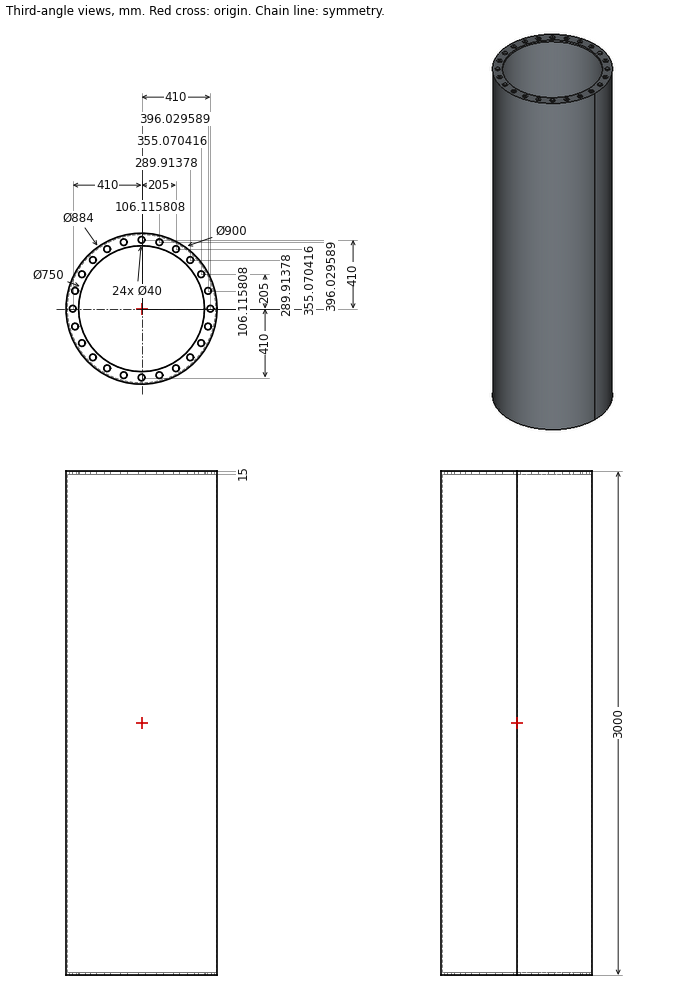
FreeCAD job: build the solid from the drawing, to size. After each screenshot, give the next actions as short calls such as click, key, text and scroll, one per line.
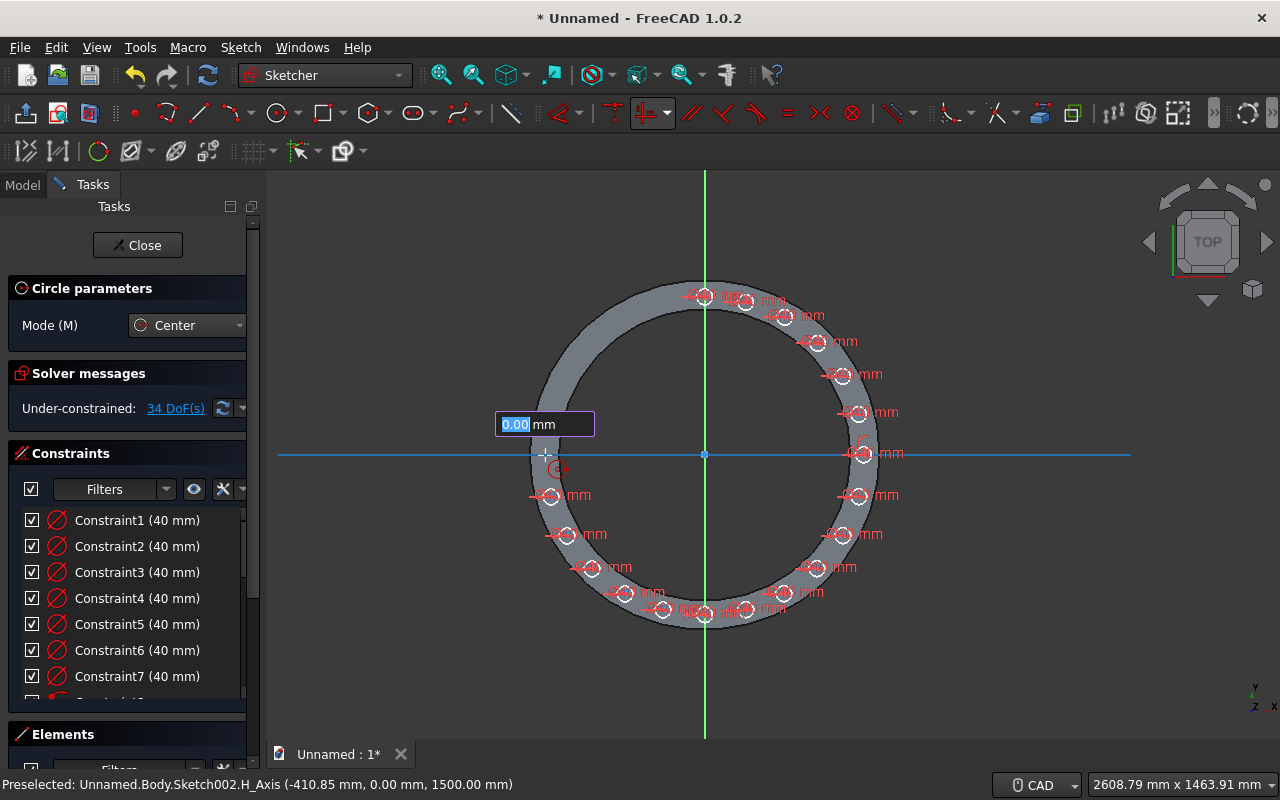
scroll(543, 462, up, 4)
move(542, 462)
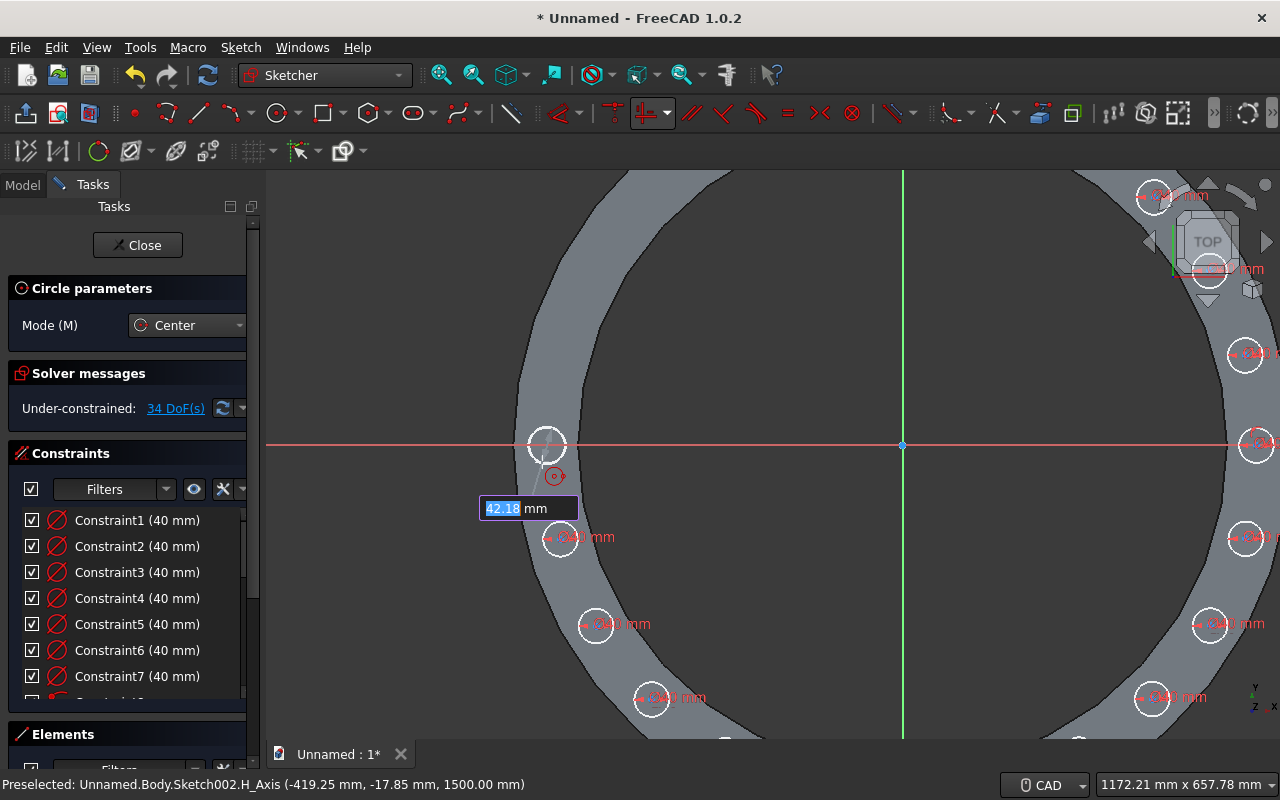
text(40)
key(Return)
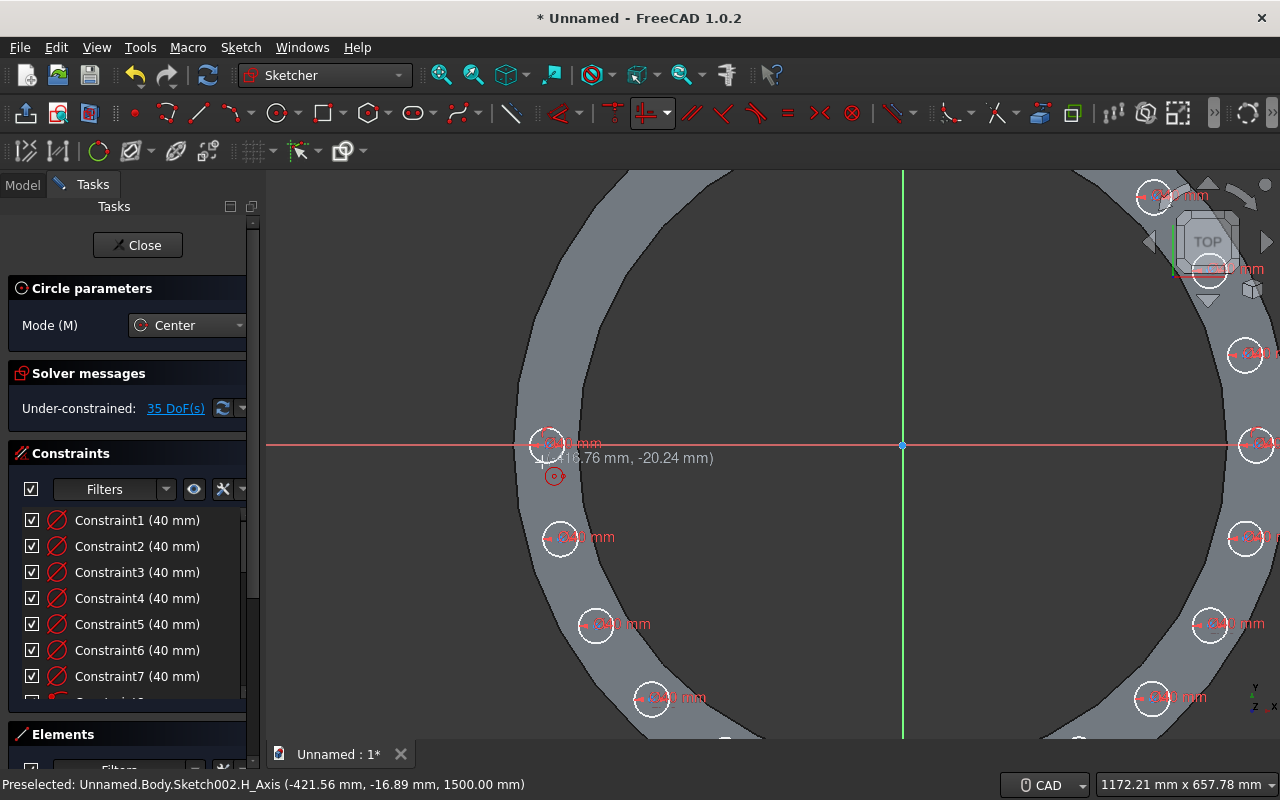
scroll(560, 354, up, 2)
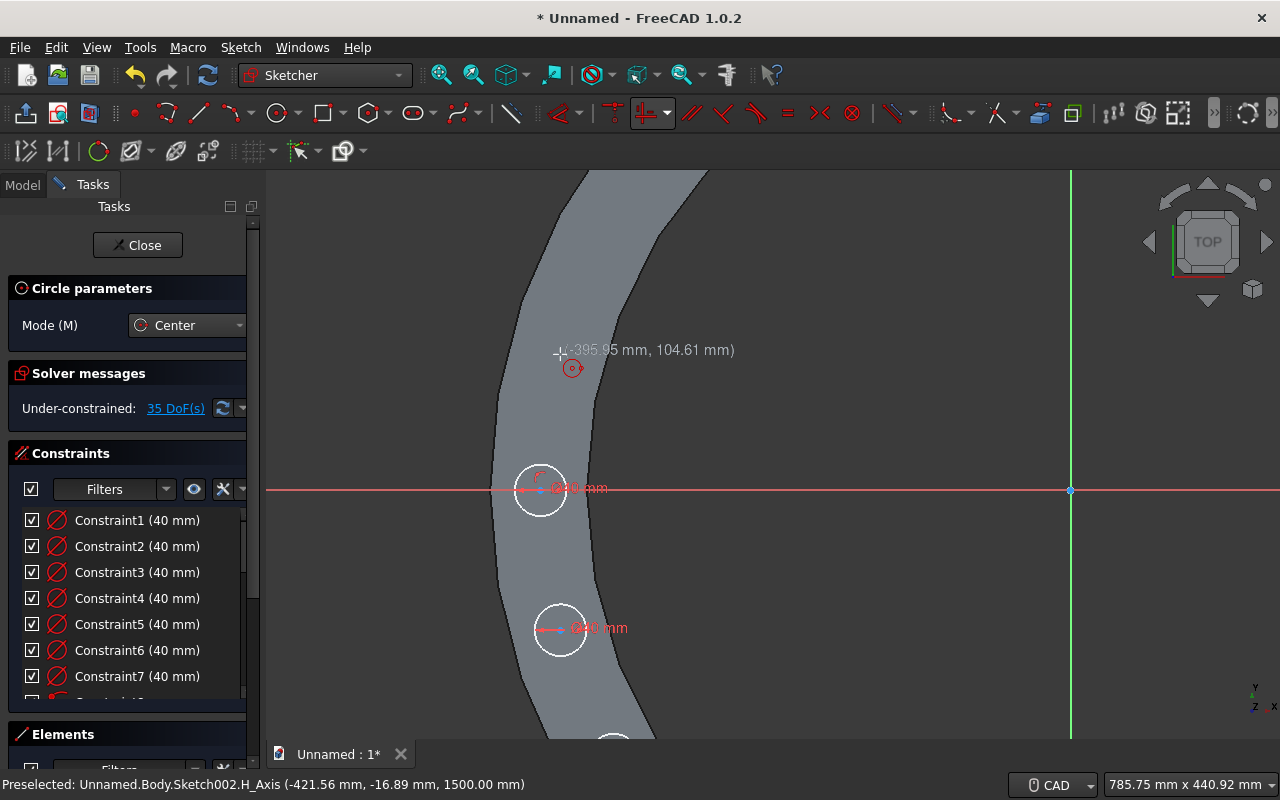
scroll(547, 439, down, 6)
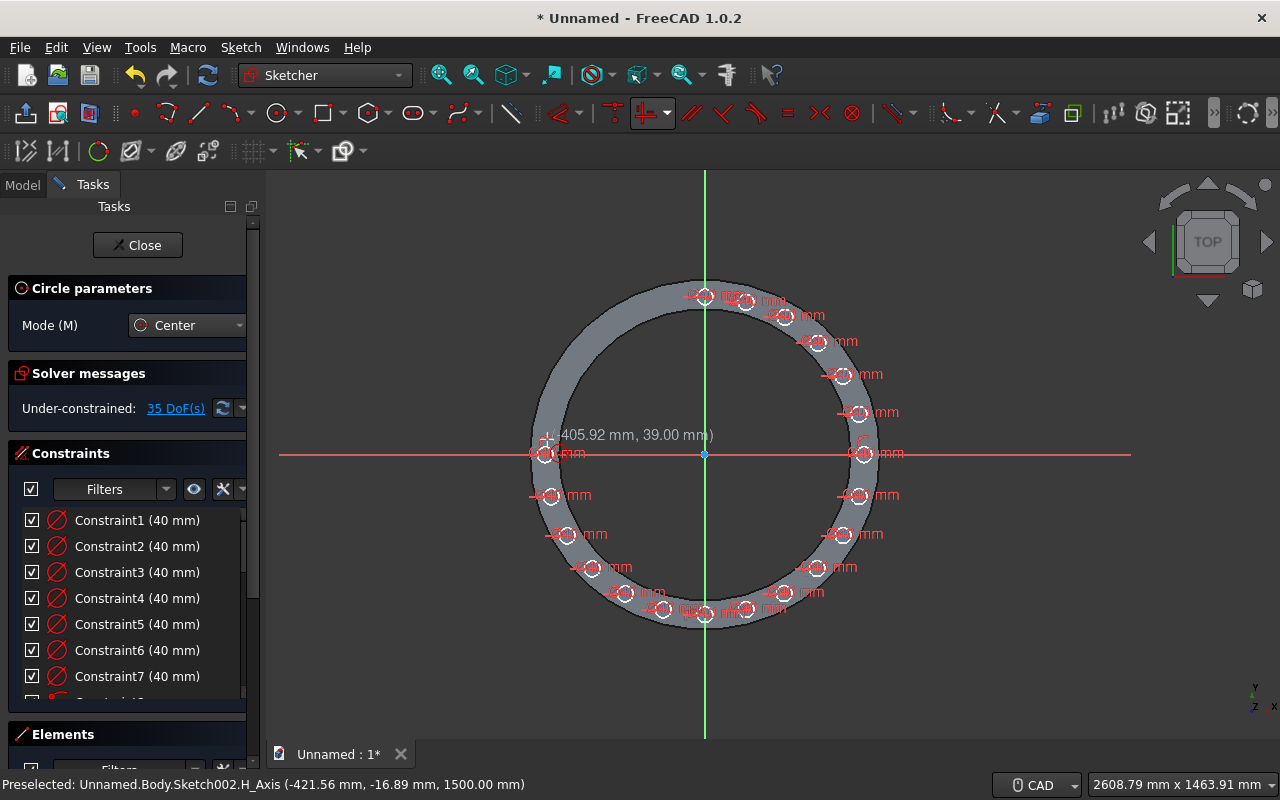
click(551, 414)
move(557, 408)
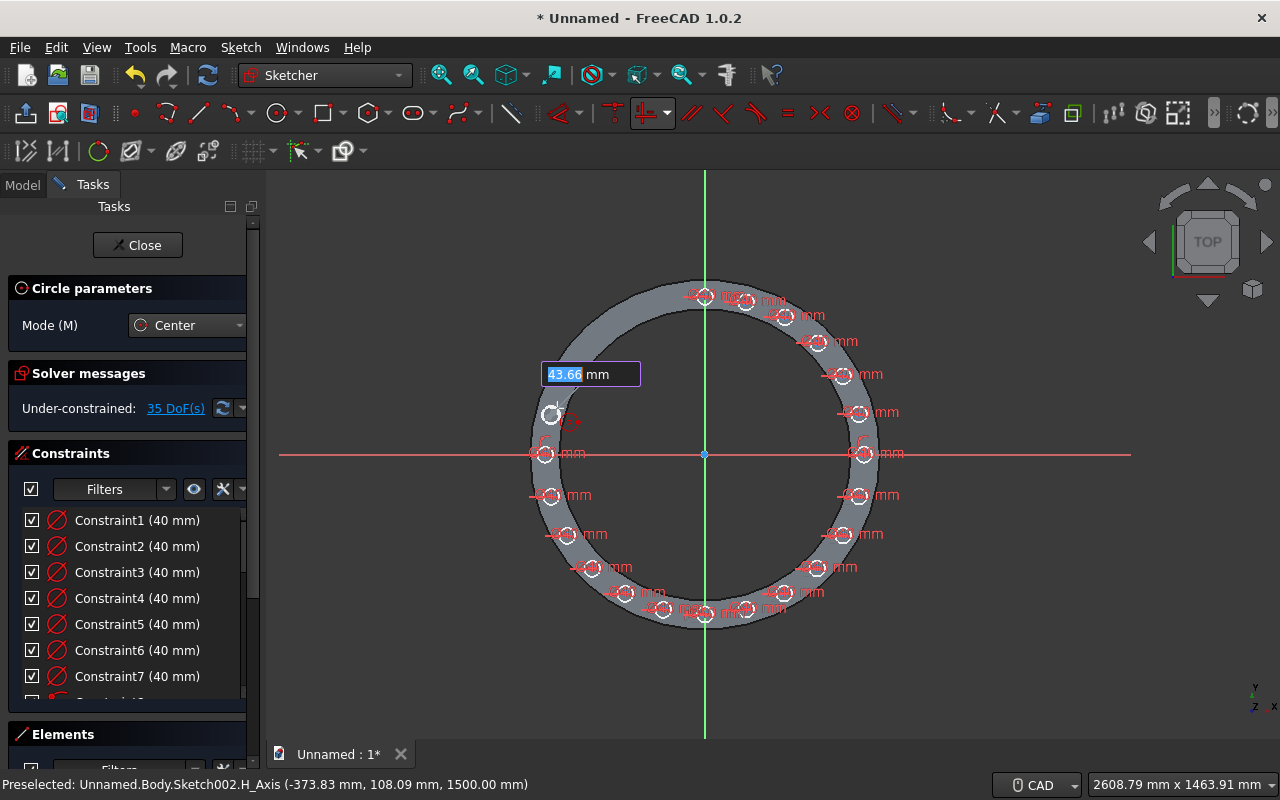
text(40)
key(Return)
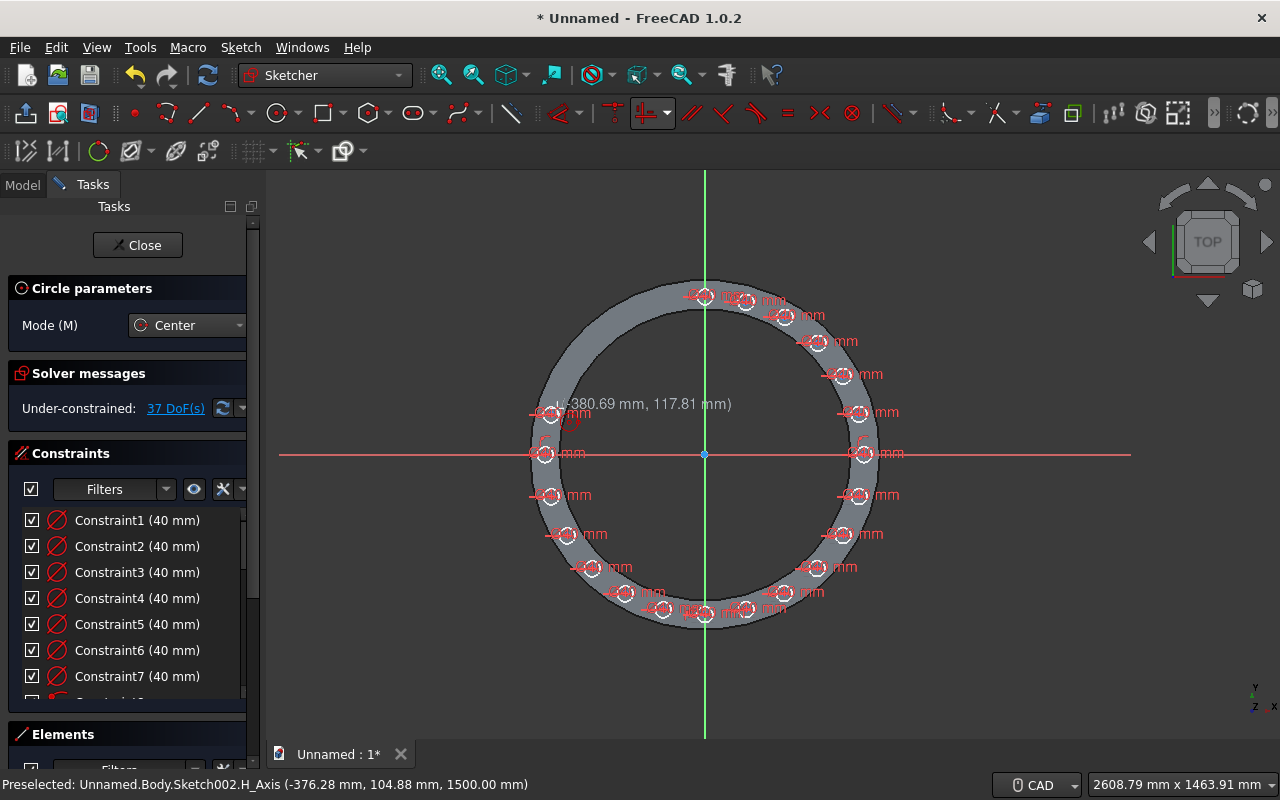
scroll(567, 375, up, 6)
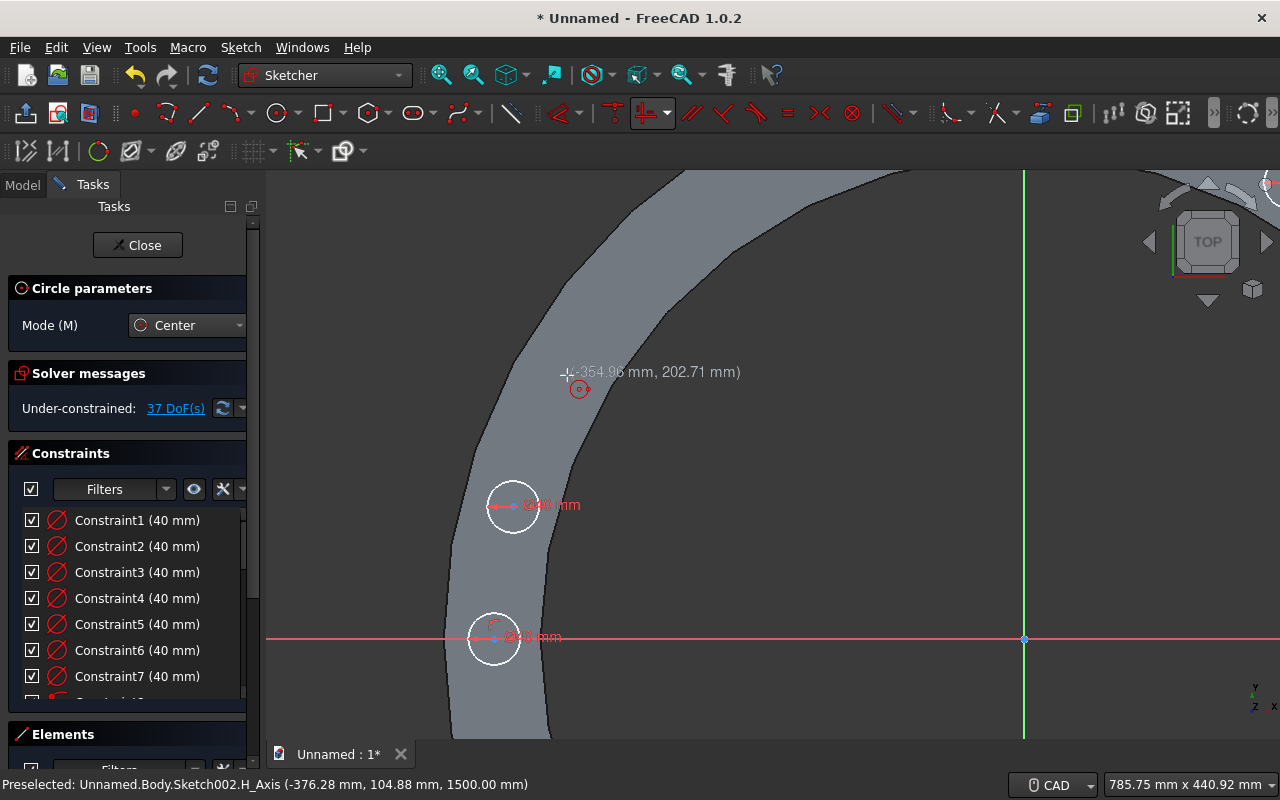
scroll(567, 375, down, 6)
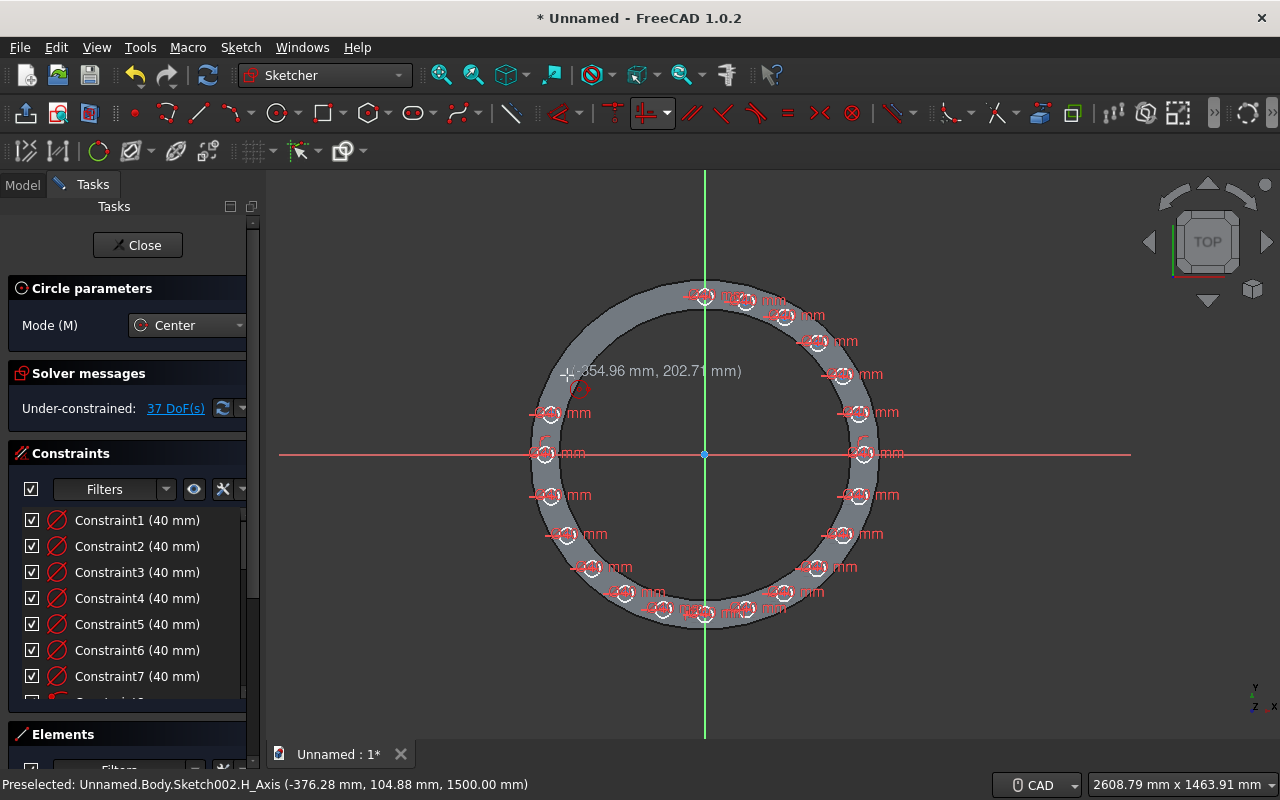
click(567, 375)
move(572, 370)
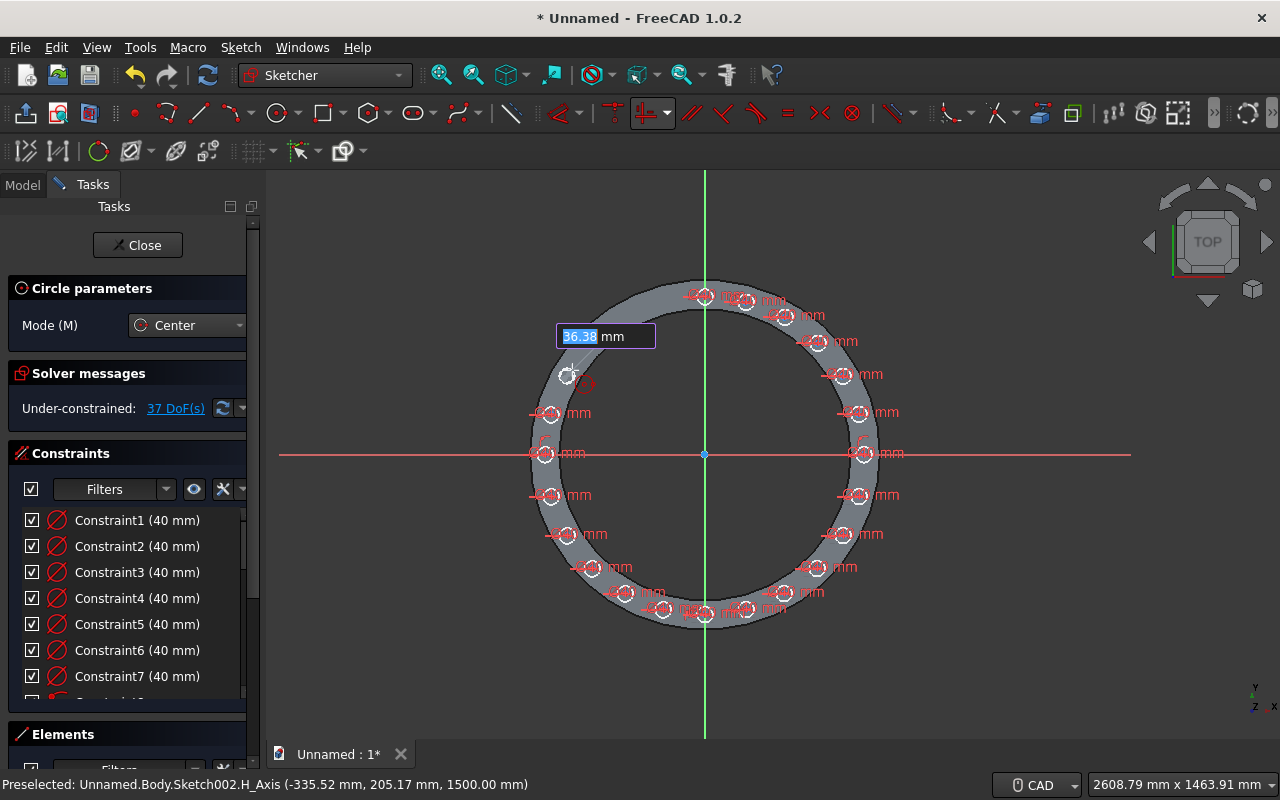
text(40)
key(Return)